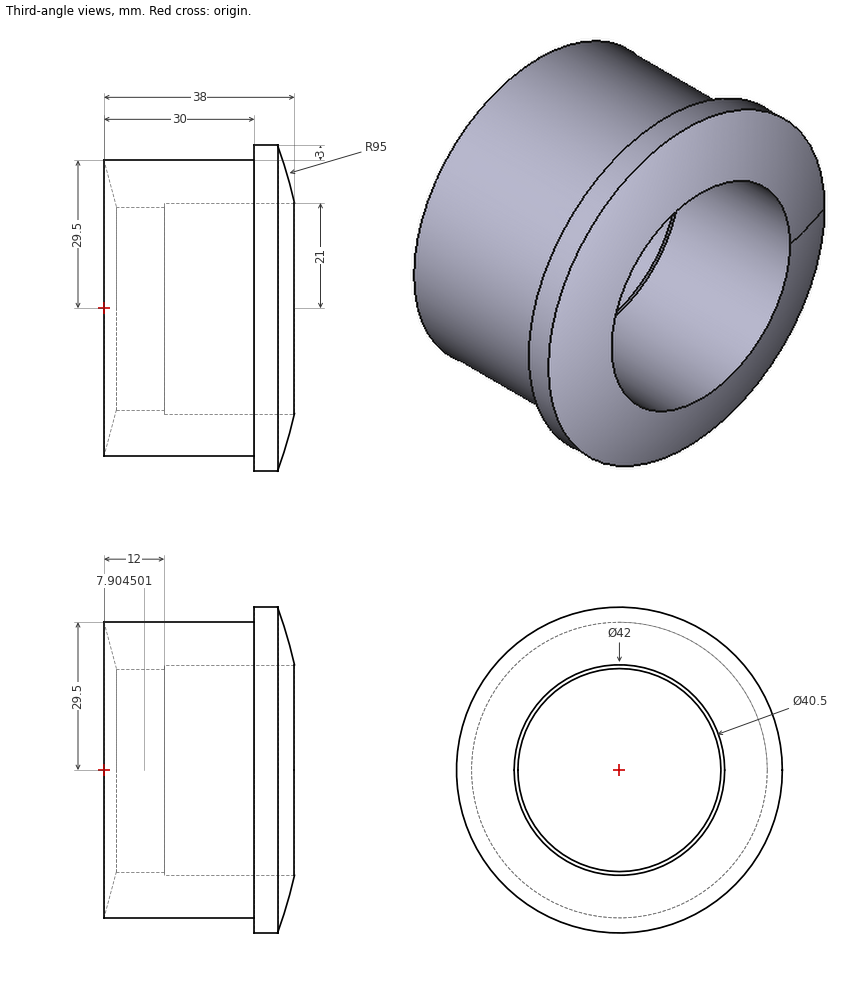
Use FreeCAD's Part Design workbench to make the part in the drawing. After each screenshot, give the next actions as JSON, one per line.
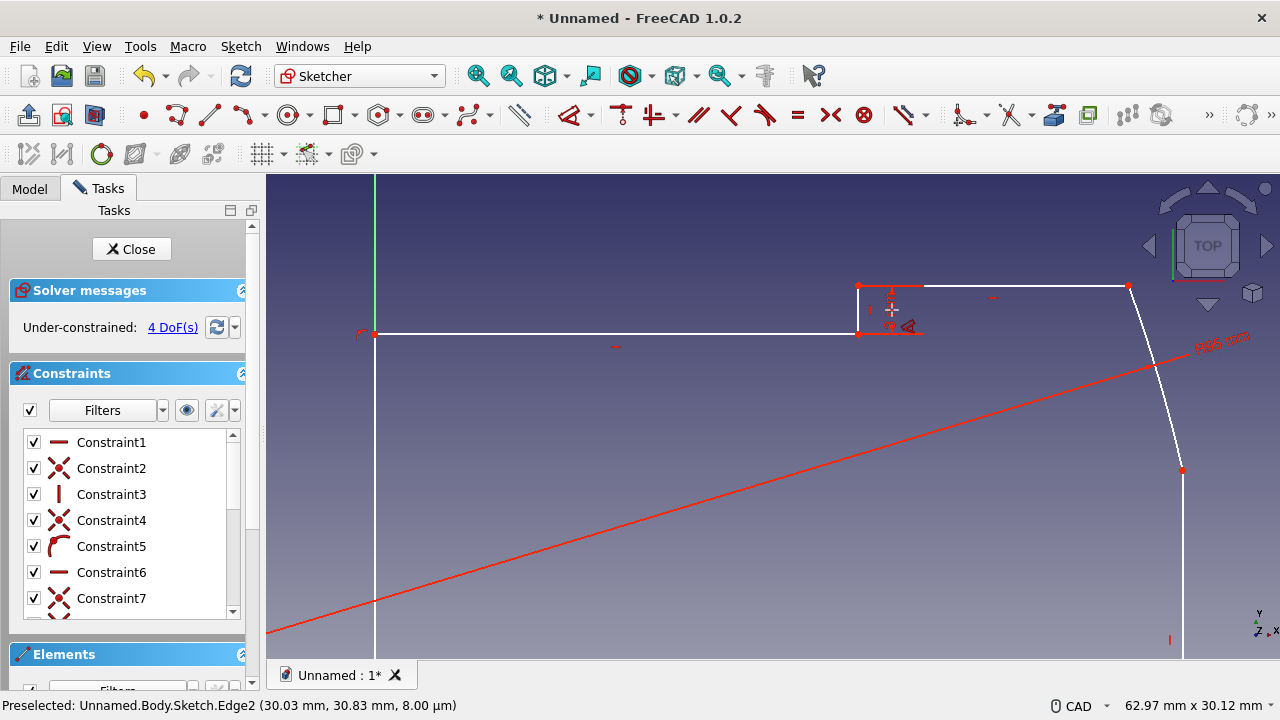
{"action": "left_click", "coordinate": [713, 334]}
{"action": "left_click", "coordinate": [616, 300]}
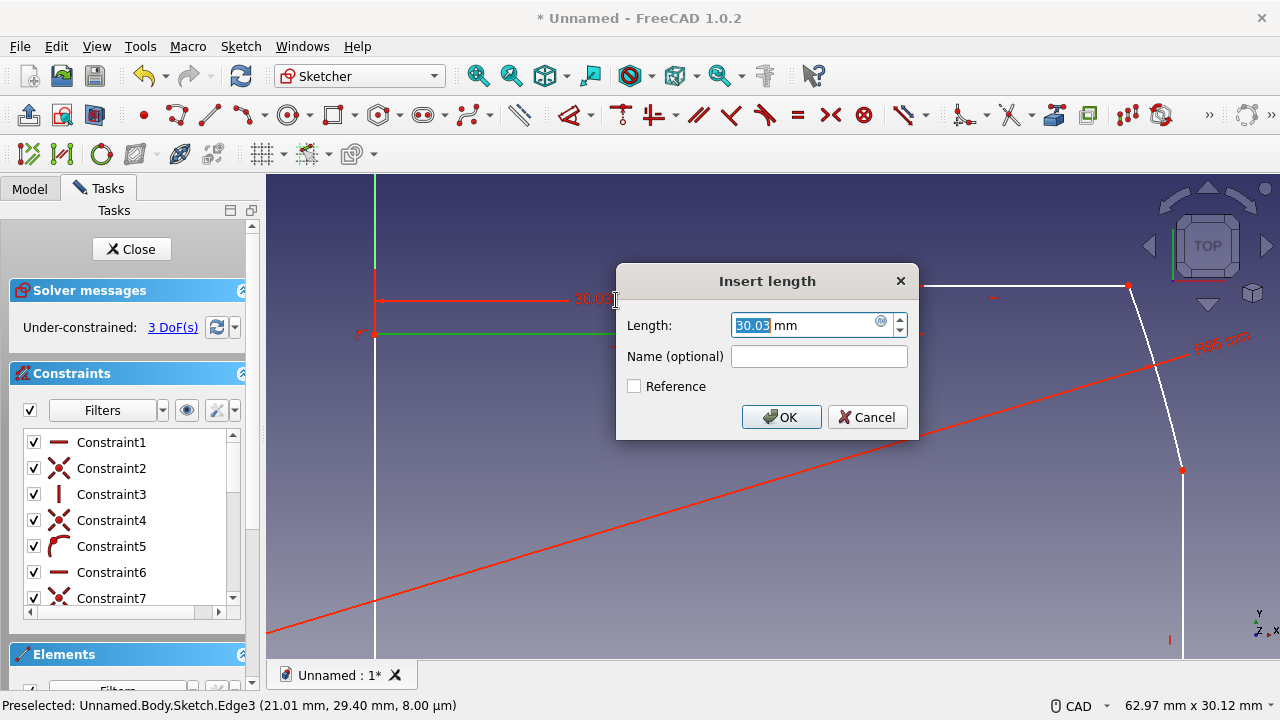
{"action": "type", "text": "30"}
{"action": "key", "text": "Return"}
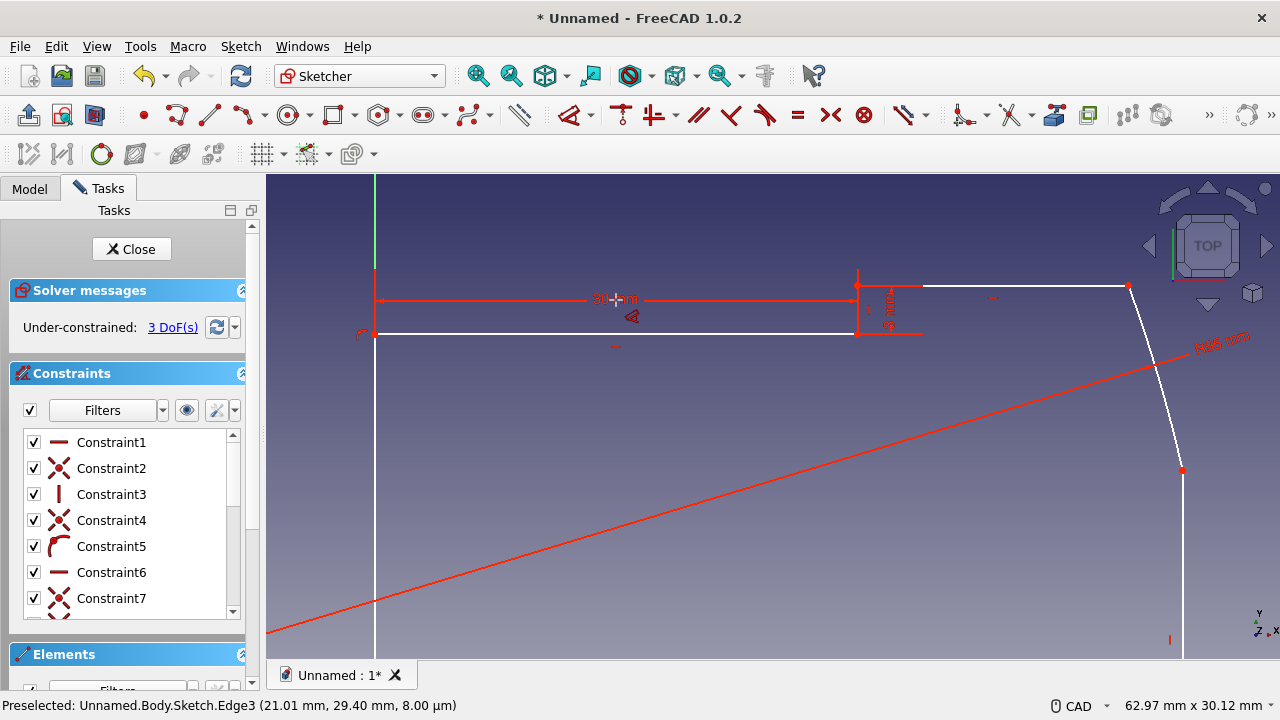
{"action": "scroll", "coordinate": [734, 259], "scroll_direction": "down", "scroll_amount": 3}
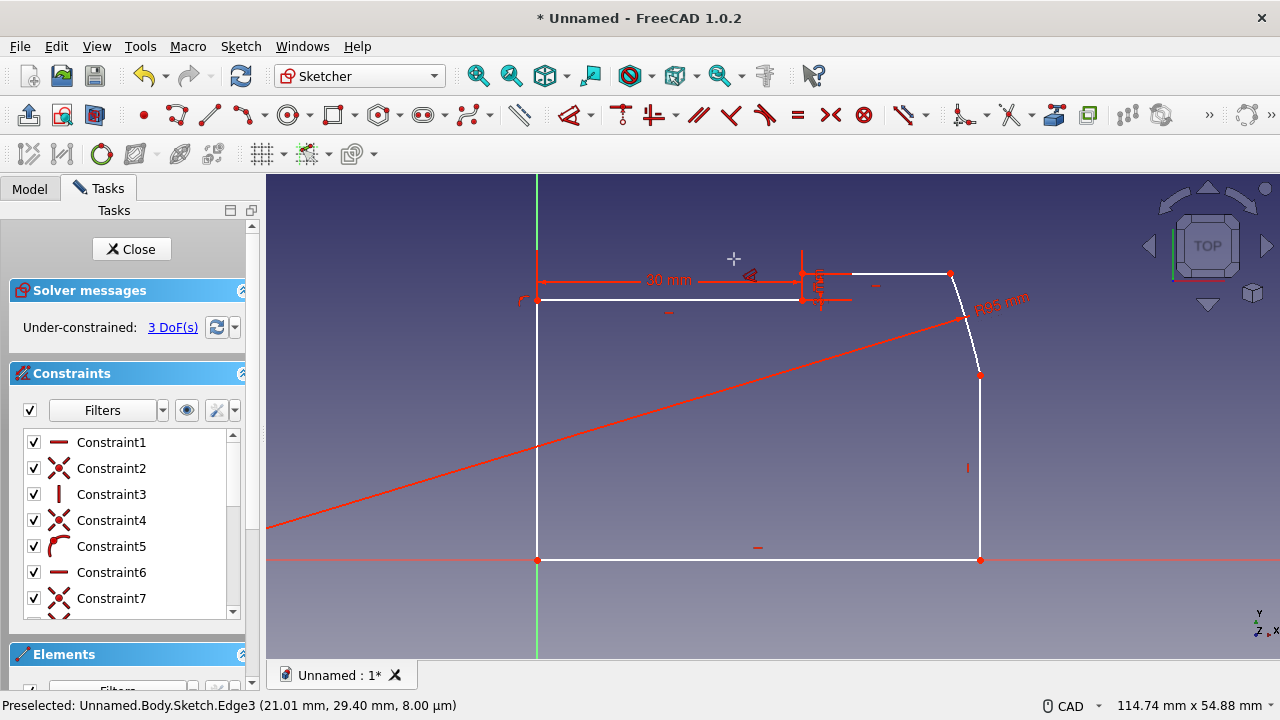
{"action": "left_click", "coordinate": [670, 560]}
{"action": "left_click", "coordinate": [759, 594]}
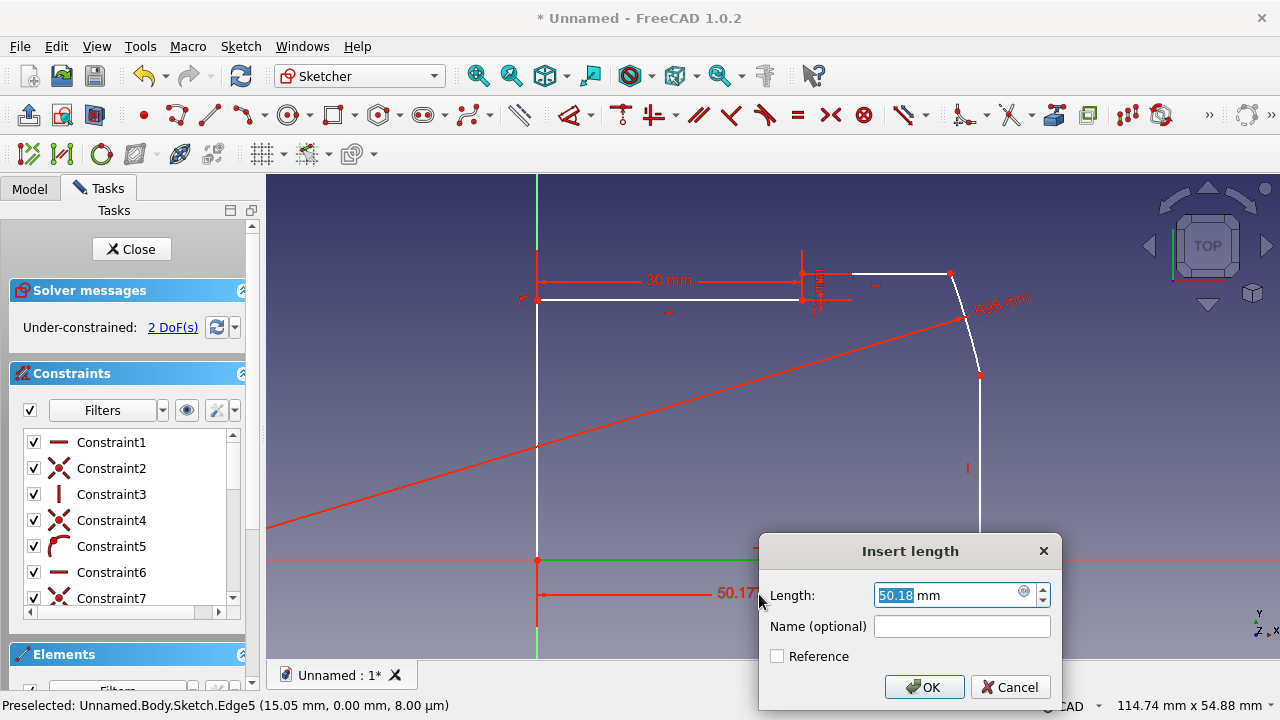
{"action": "type", "text": "38"}
{"action": "key", "text": "Return"}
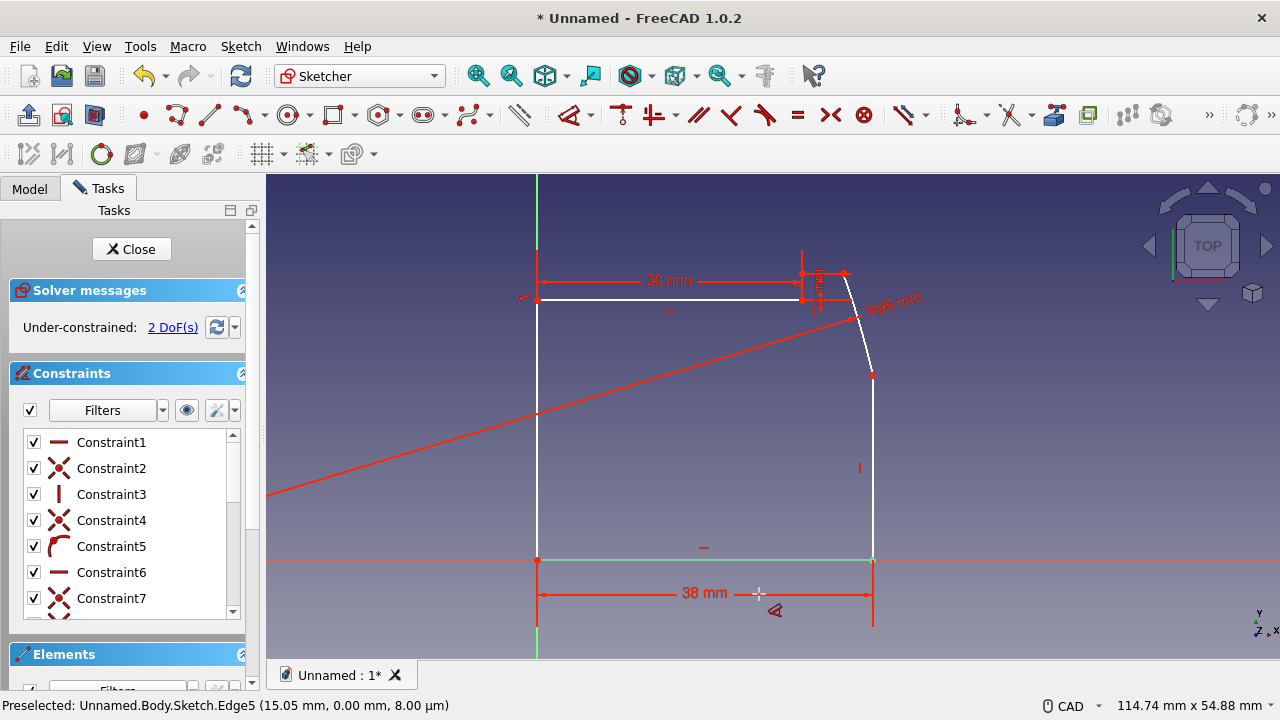
{"action": "left_click", "coordinate": [873, 505]}
{"action": "left_click", "coordinate": [907, 468]}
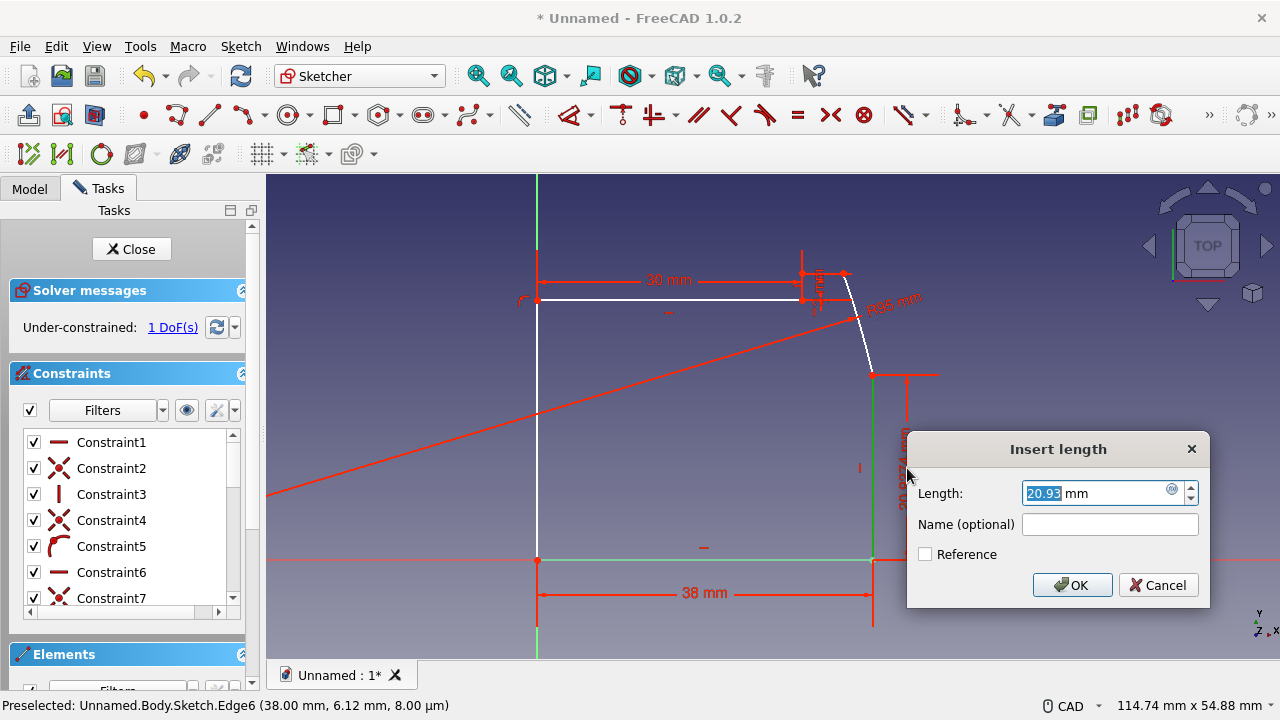
{"action": "type", "text": "21"}
{"action": "key", "text": "Return"}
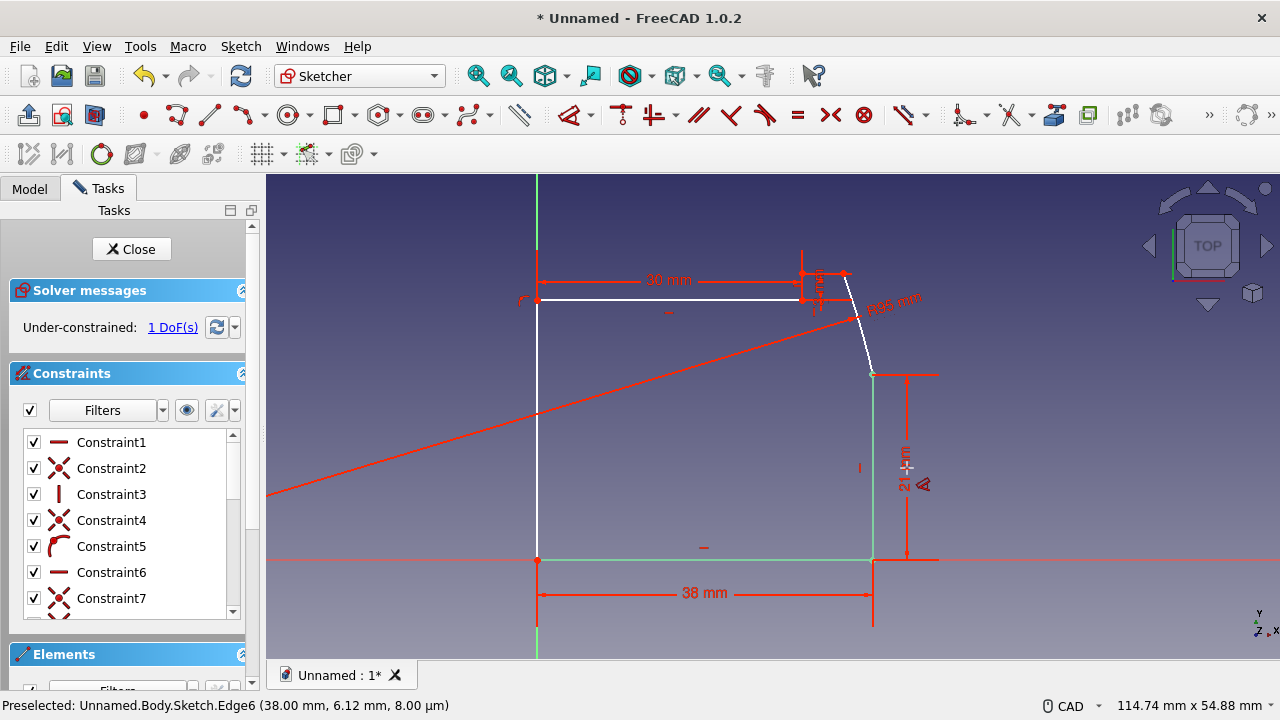
{"action": "left_click", "coordinate": [537, 378]}
{"action": "left_click", "coordinate": [503, 430]}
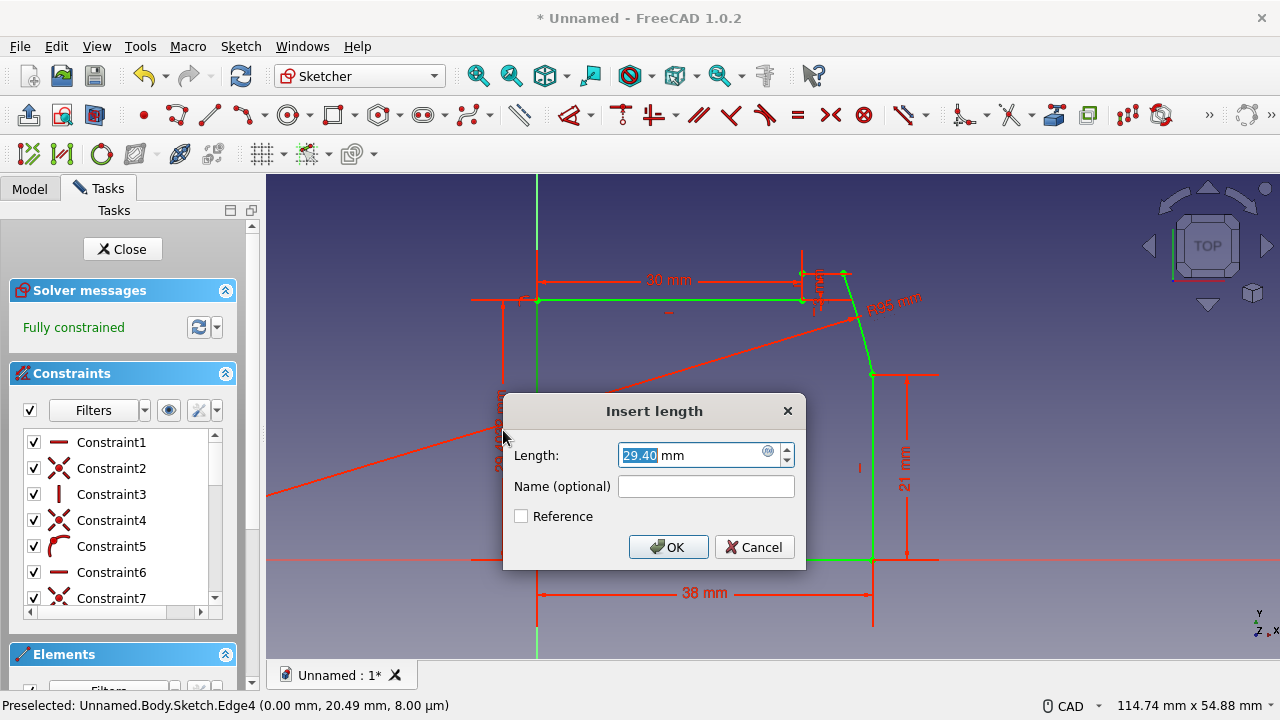
{"action": "type", "text": "29.5"}
{"action": "key", "text": "Return"}
{"action": "key", "text": "Escape"}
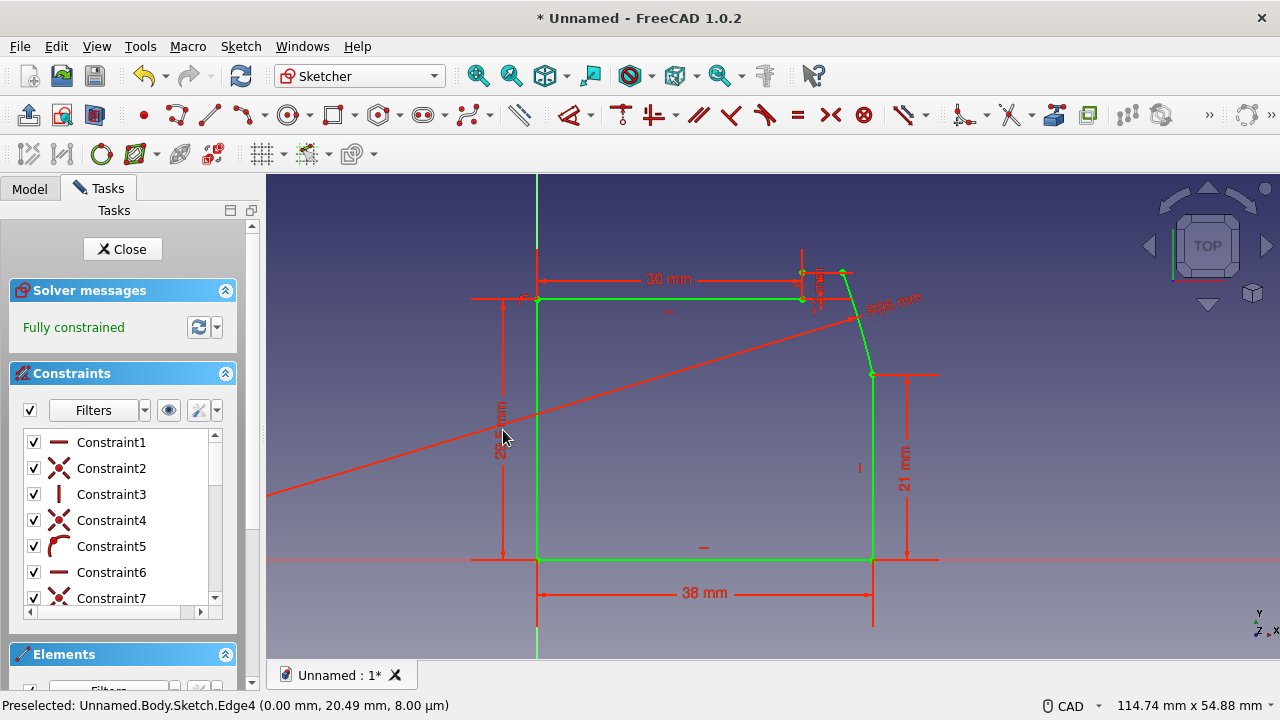
{"action": "left_click", "coordinate": [123, 249]}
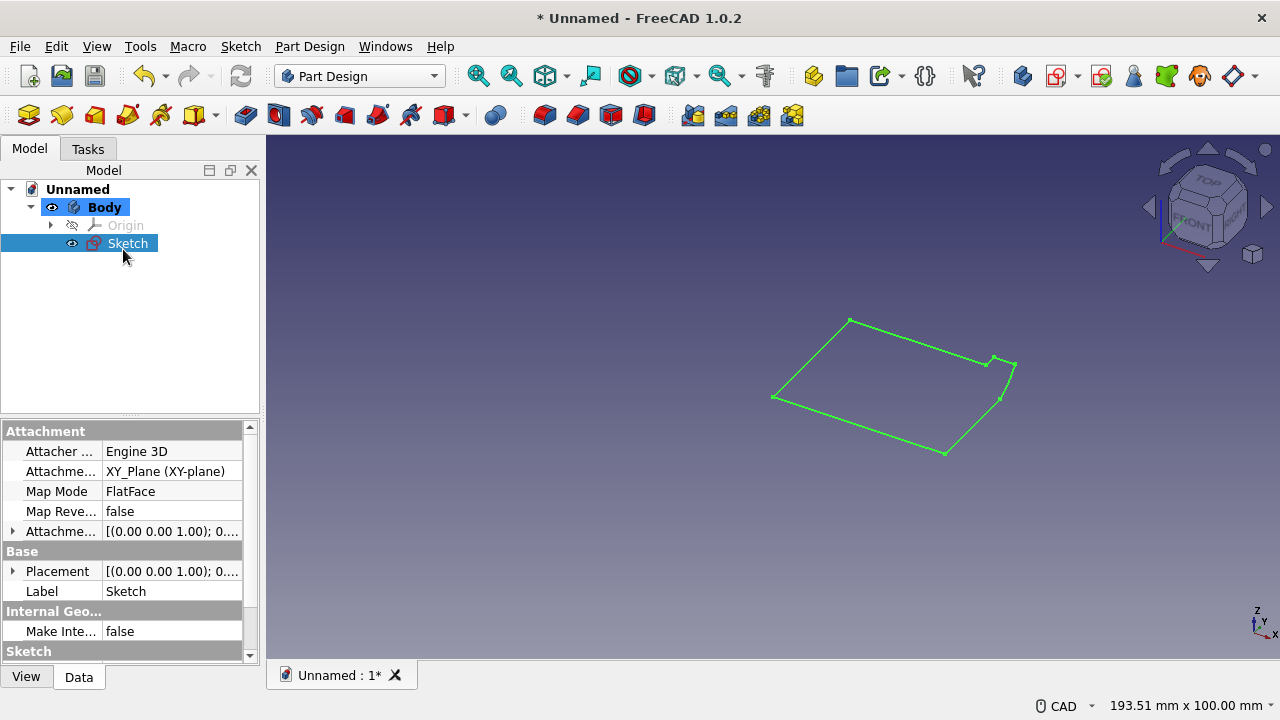
{"action": "left_click", "coordinate": [62, 116]}